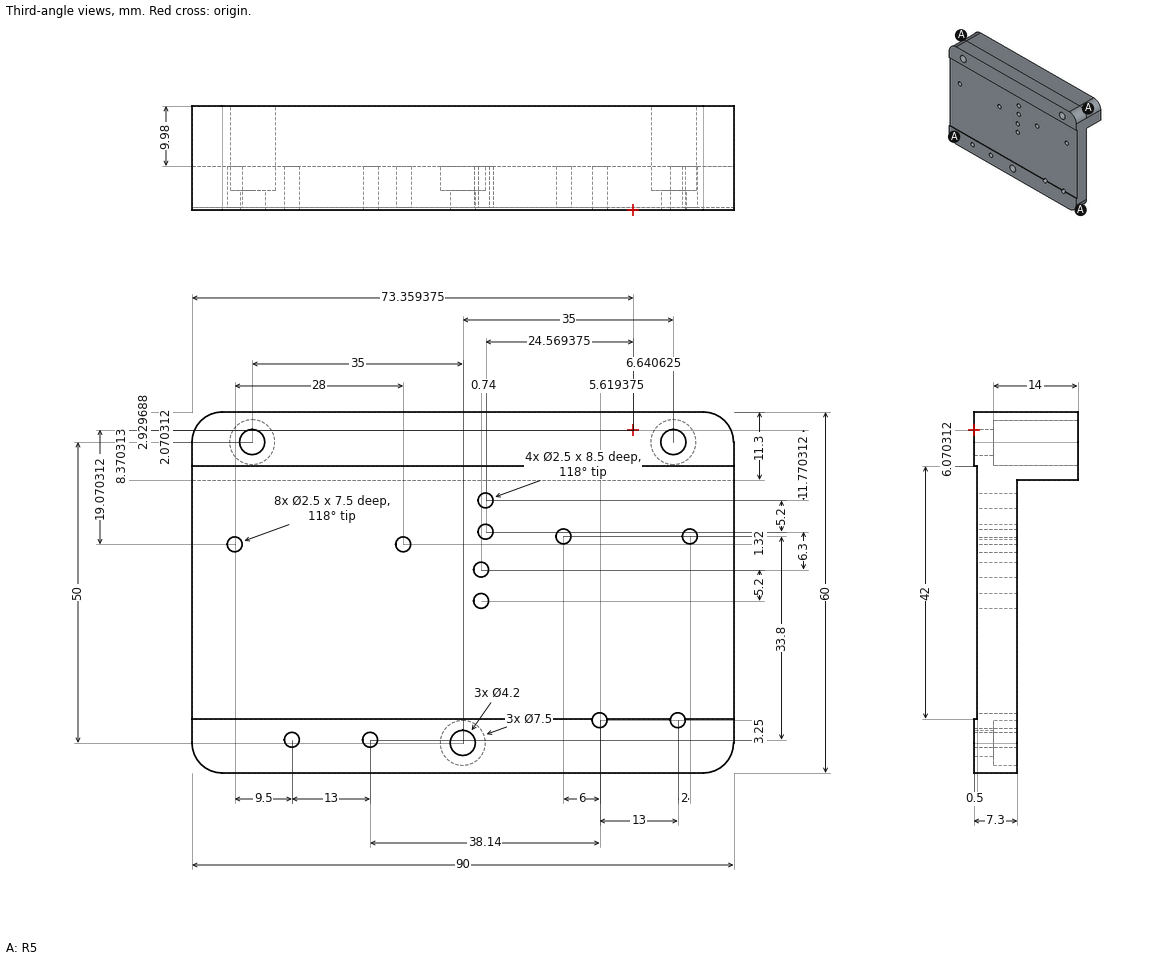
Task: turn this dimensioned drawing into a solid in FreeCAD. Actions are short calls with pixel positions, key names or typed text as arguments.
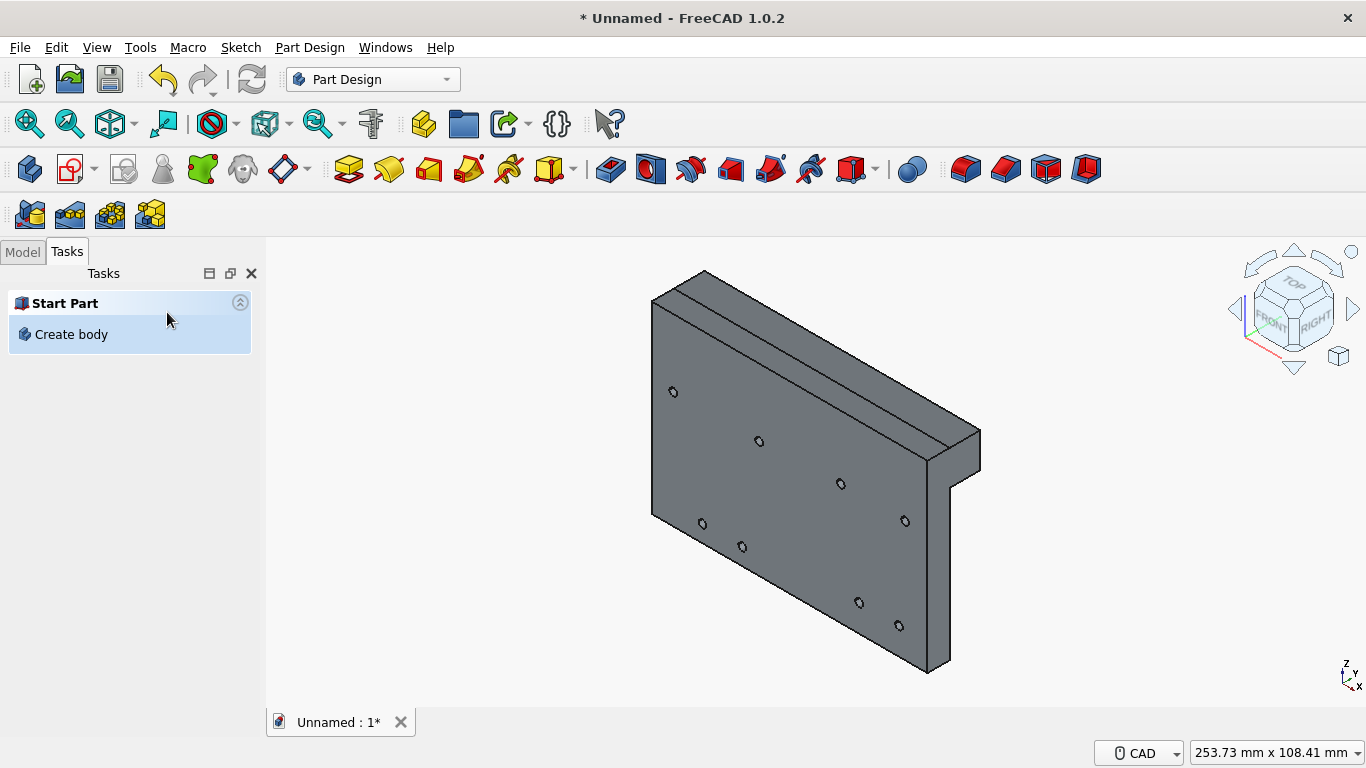
click(965, 438)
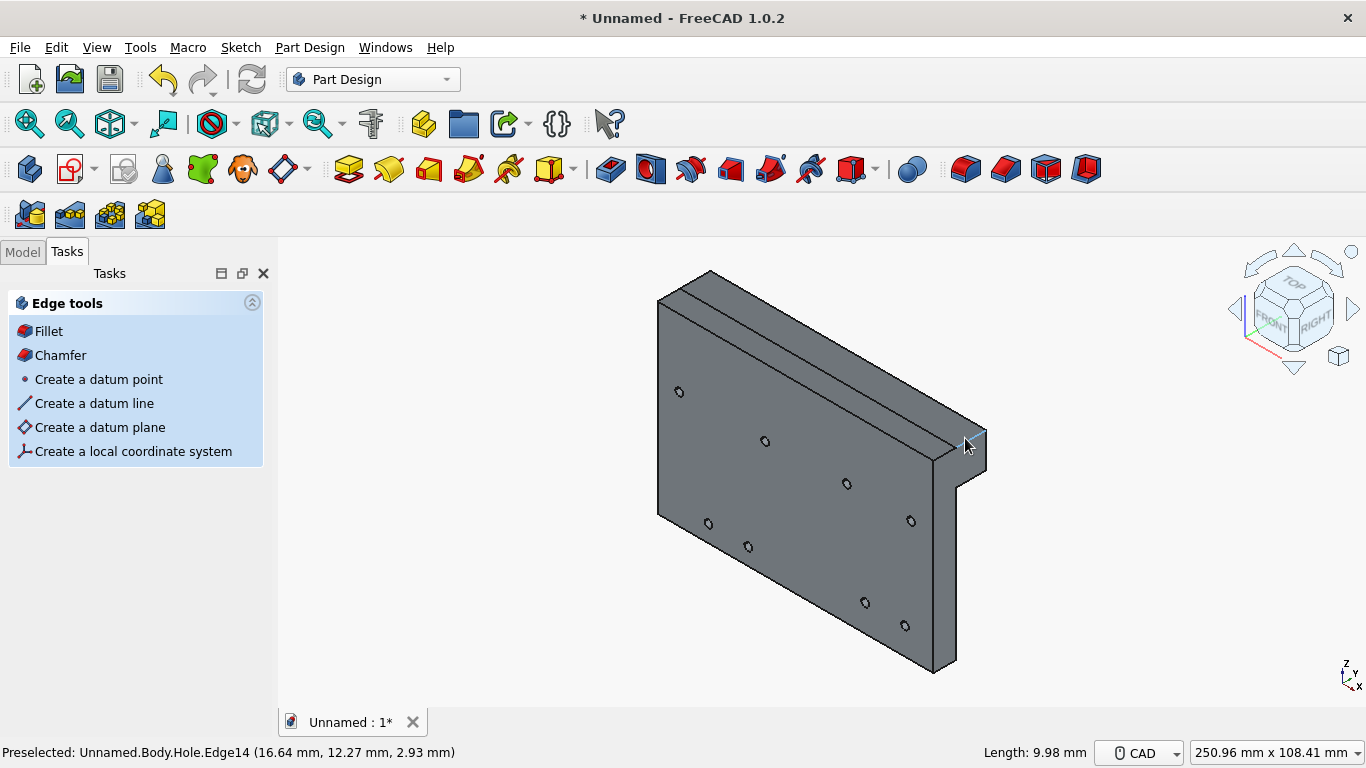
key(2)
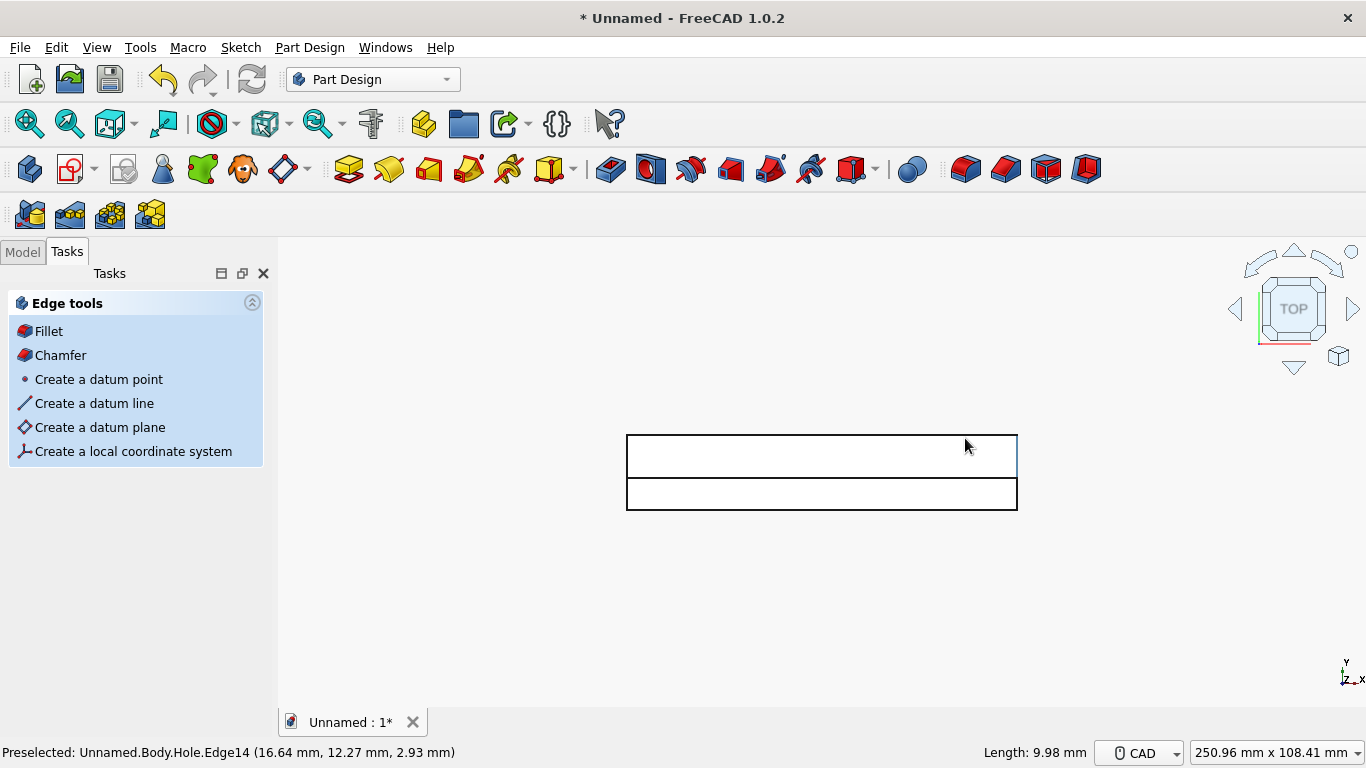
click(30, 124)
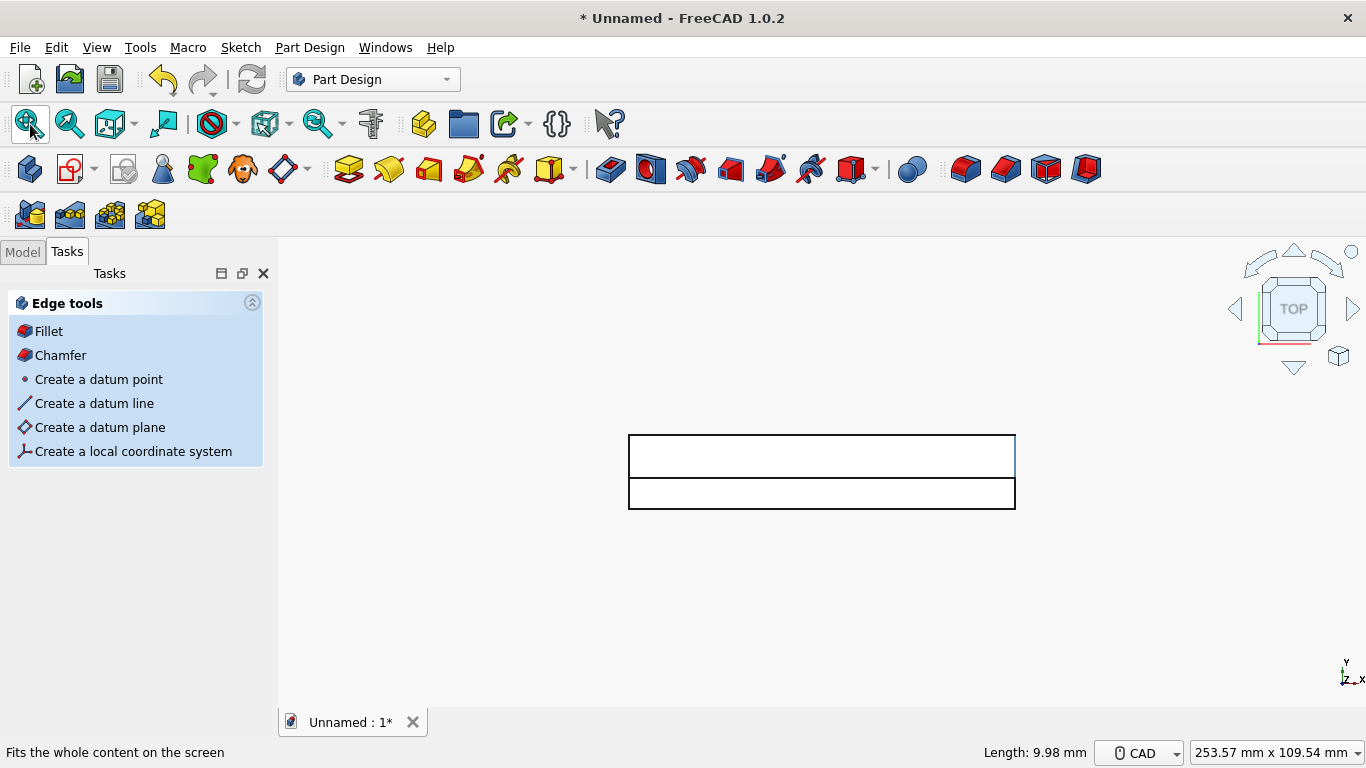
click(629, 455, ctrl)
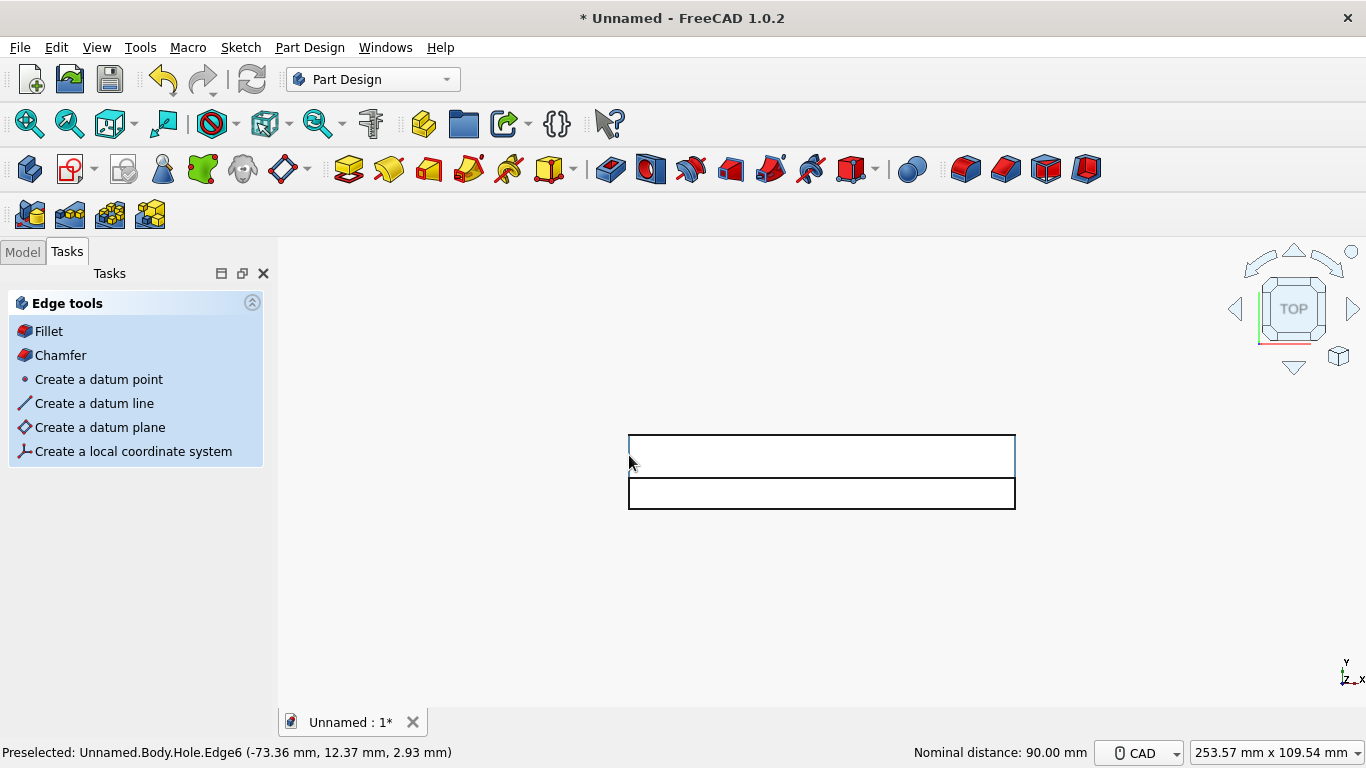
key(1)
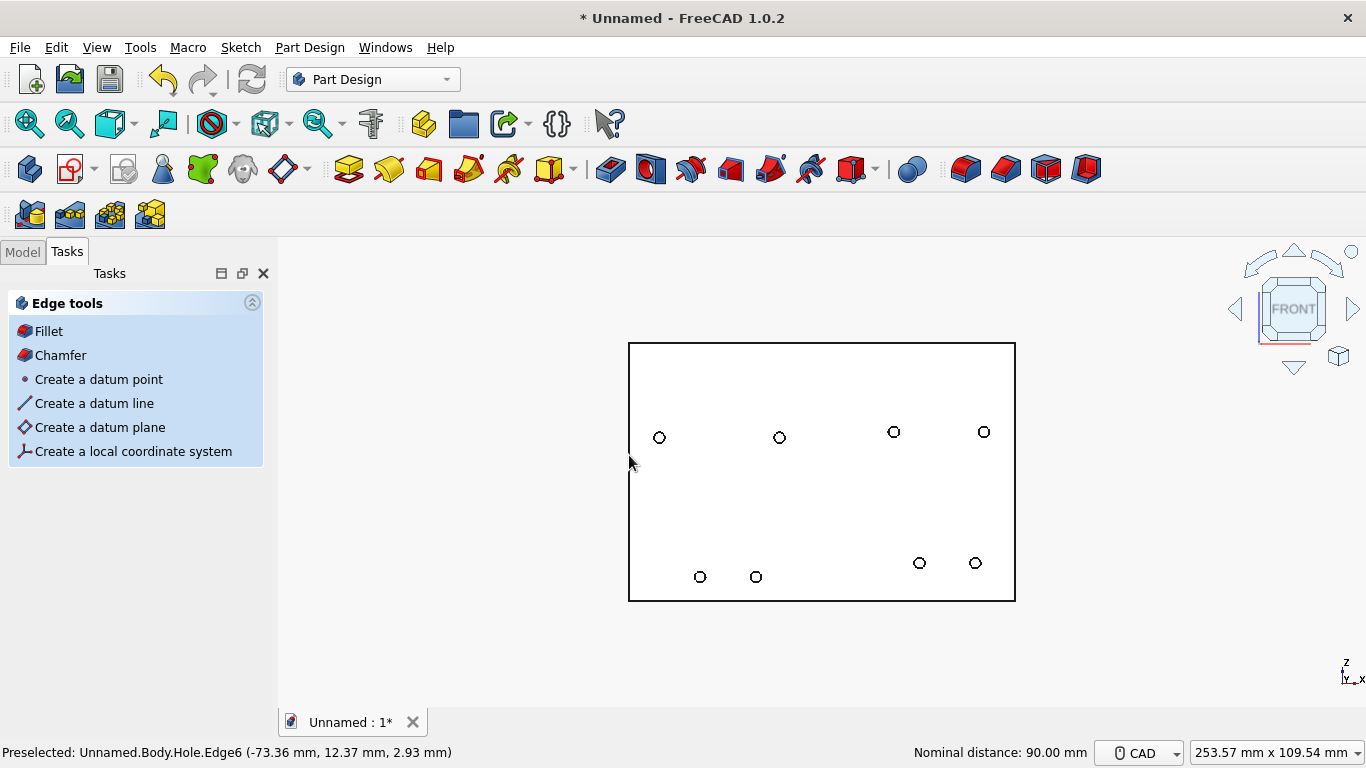
key(3)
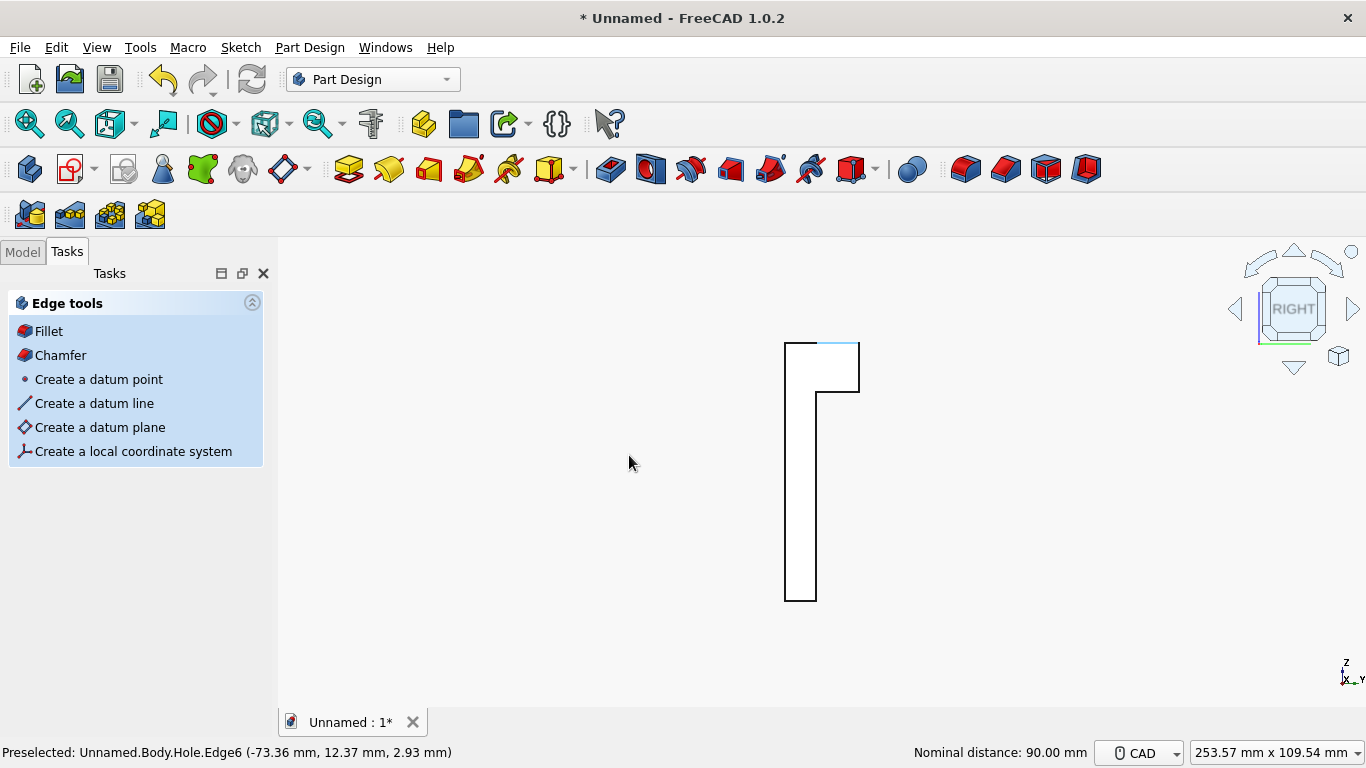
click(801, 600, ctrl)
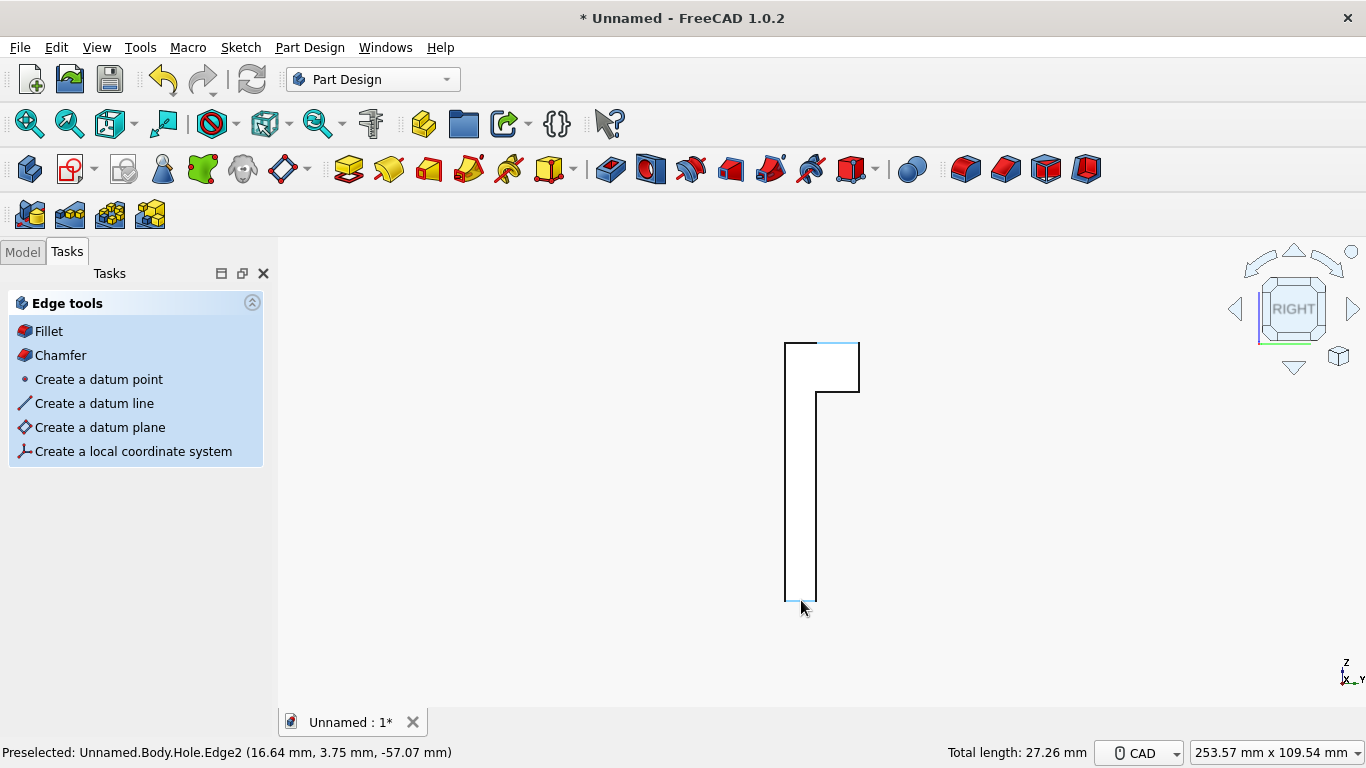
key(5)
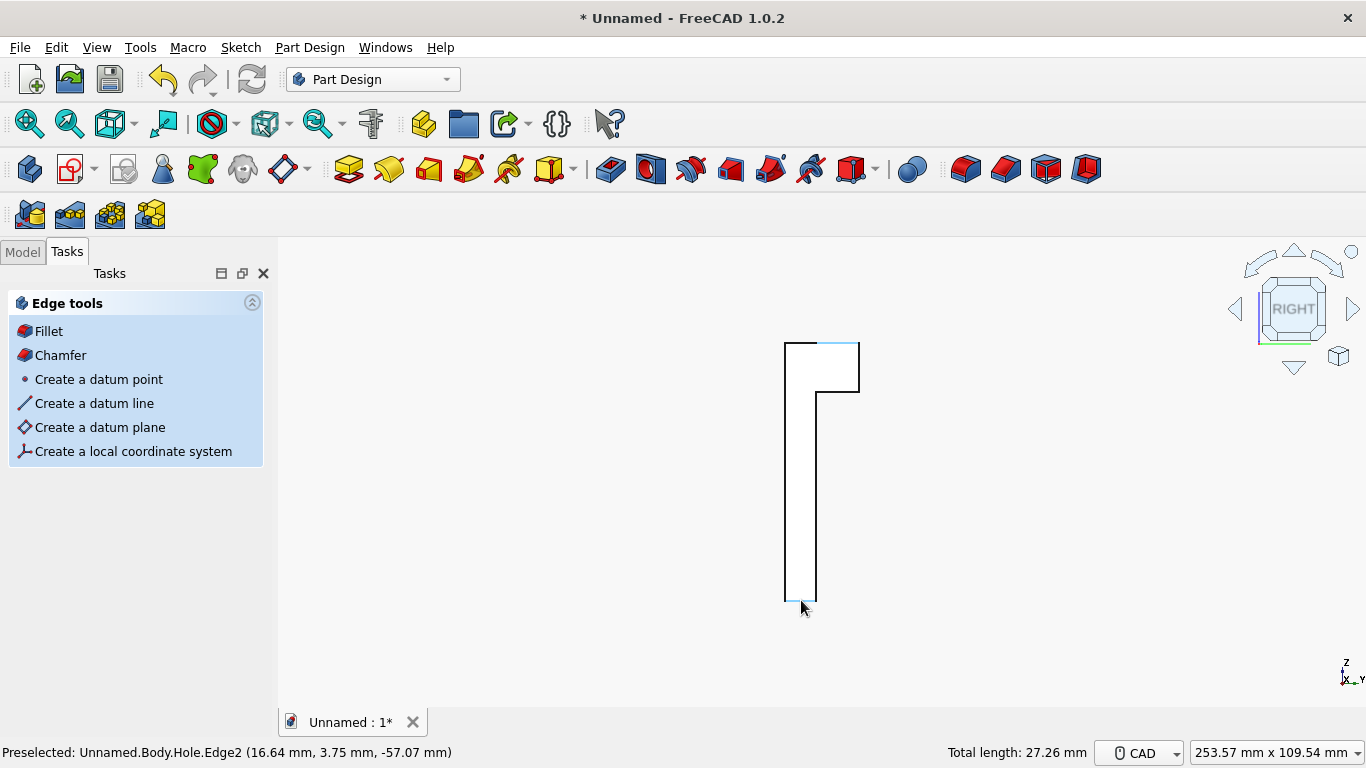
click(30, 124)